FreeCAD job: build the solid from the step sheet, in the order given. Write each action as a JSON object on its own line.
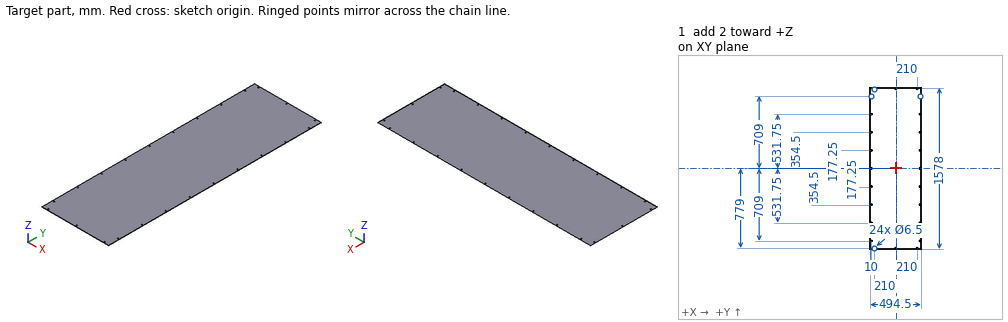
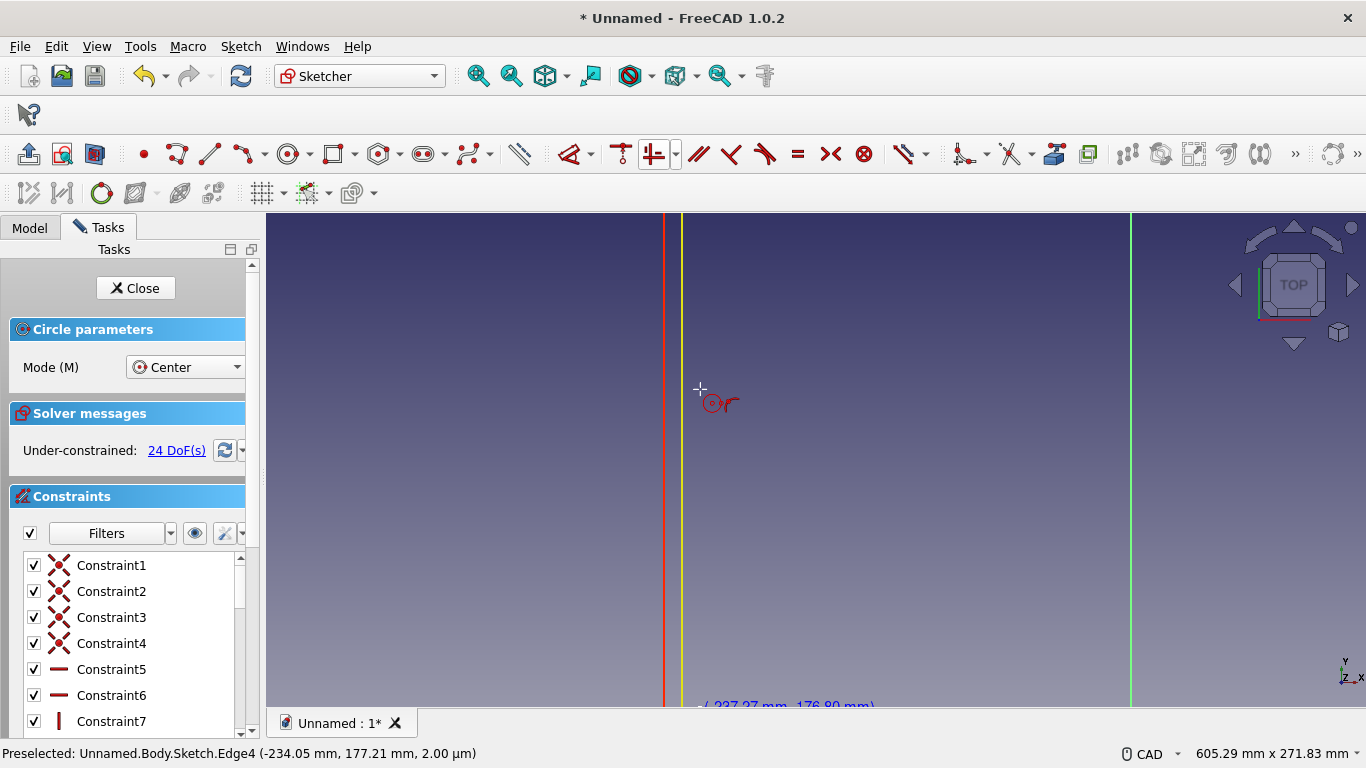
{"action": "left_click", "coordinate": [700, 390]}
{"action": "mouse_move", "coordinate": [704, 385]}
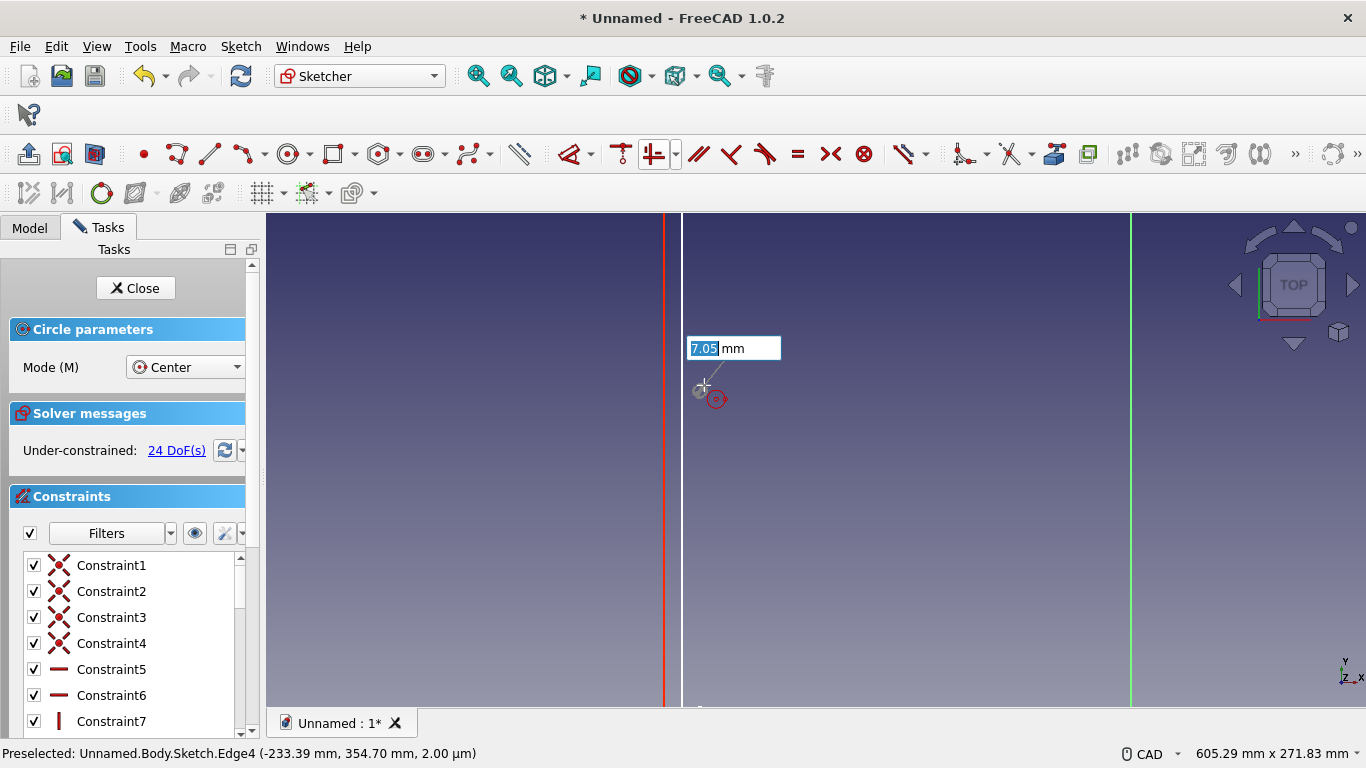
{"action": "type", "text": "6.5"}
{"action": "key", "text": "Return"}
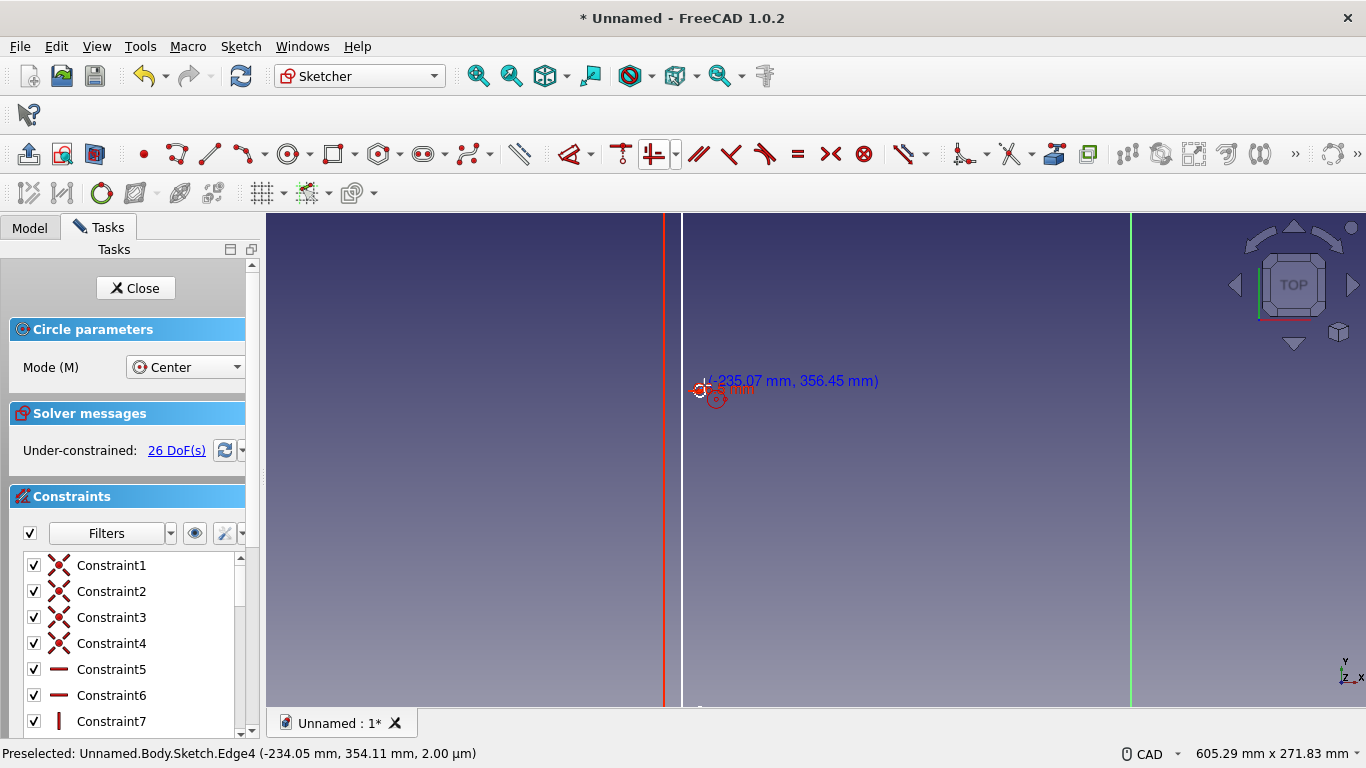
{"action": "scroll", "coordinate": [700, 389], "scroll_direction": "down", "scroll_amount": 11}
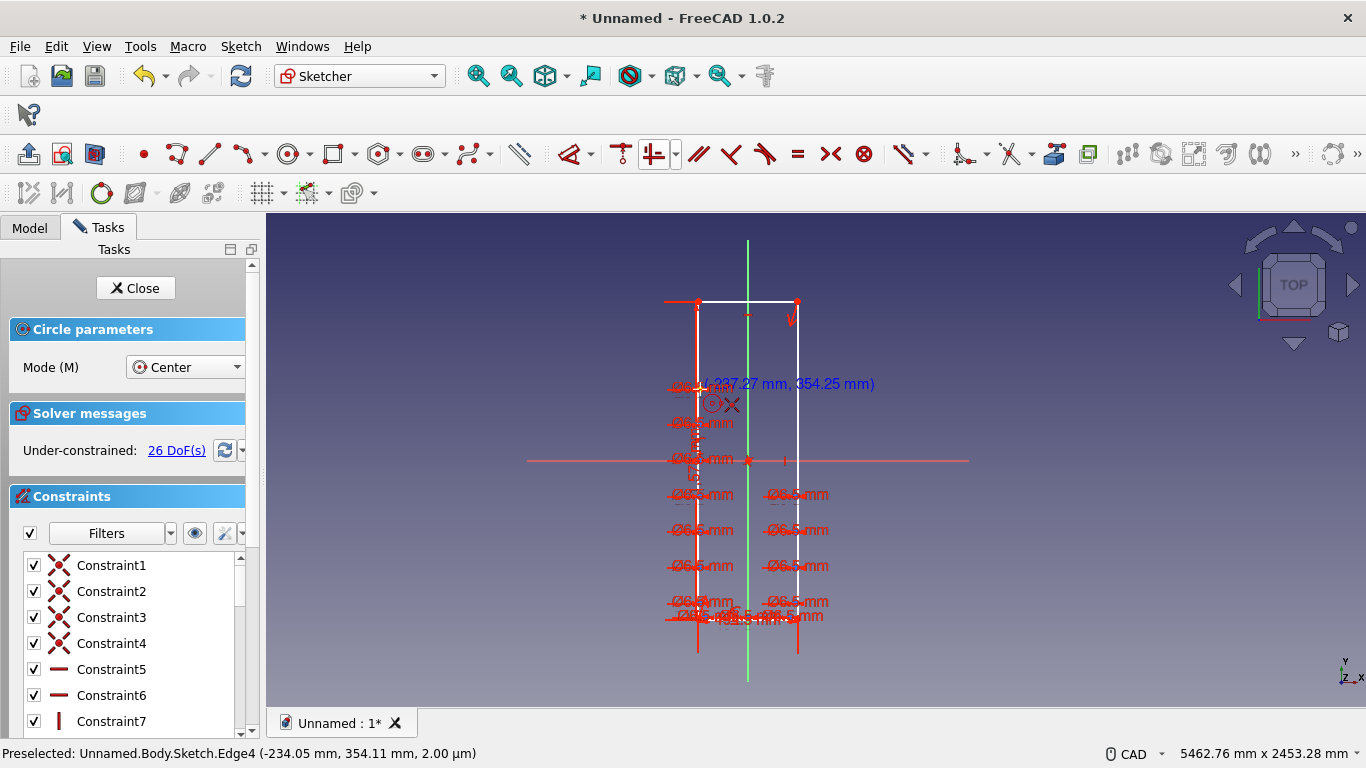
{"action": "scroll", "coordinate": [700, 354], "scroll_direction": "up", "scroll_amount": 18}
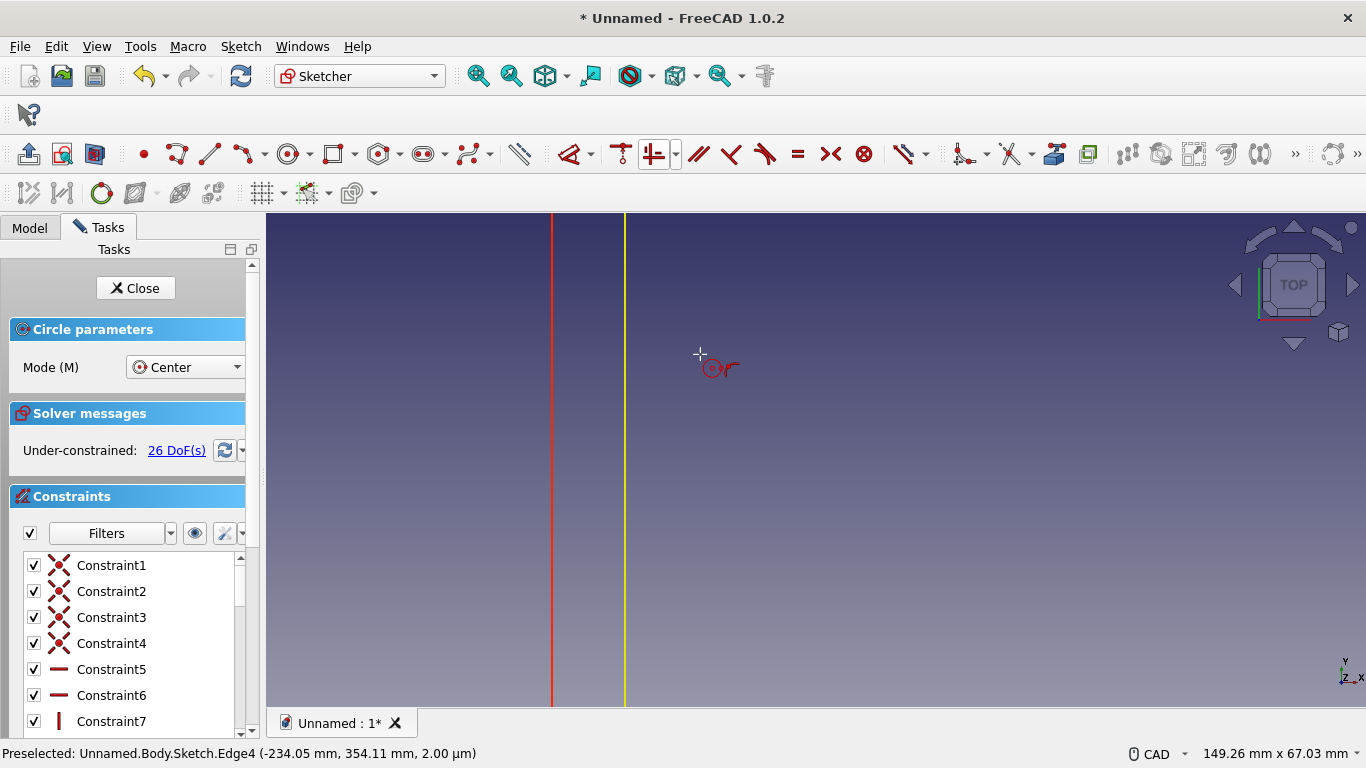
{"action": "scroll", "coordinate": [700, 354], "scroll_direction": "down", "scroll_amount": 18}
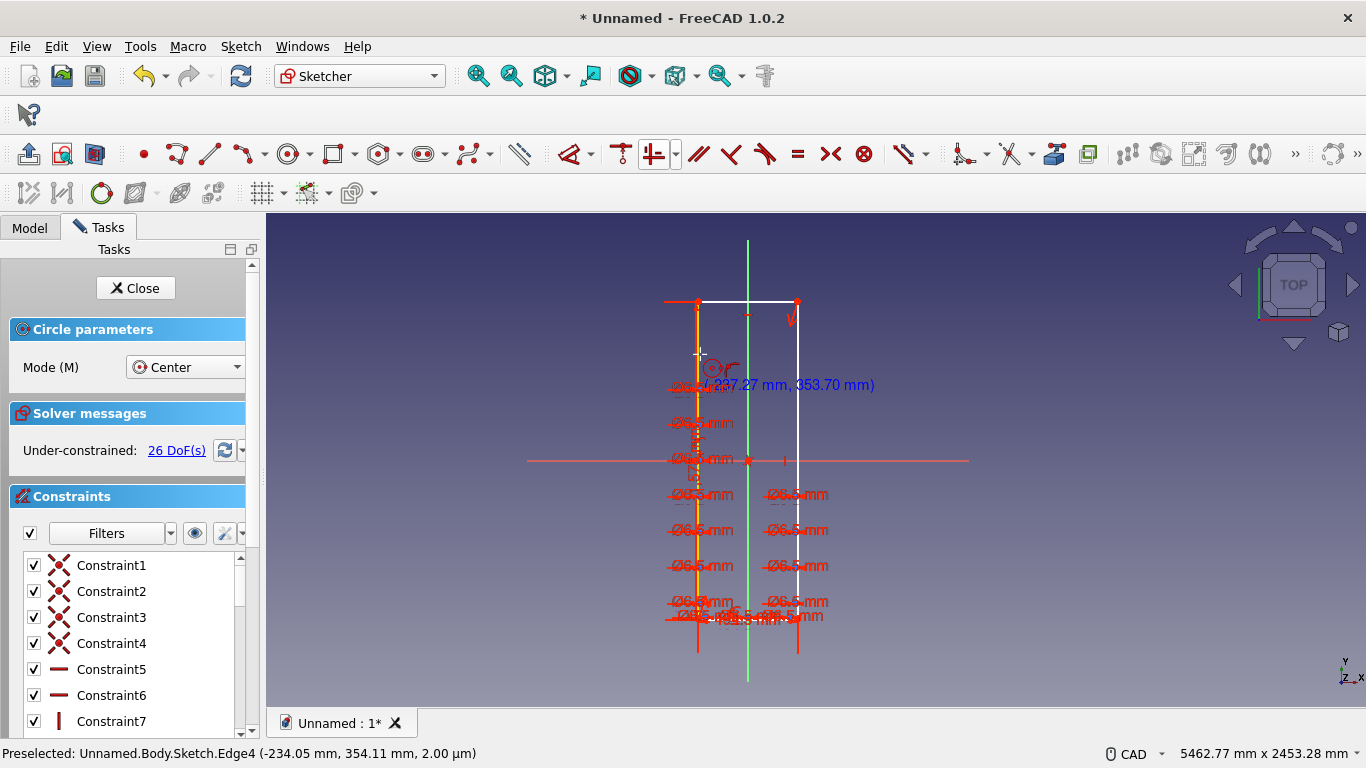
{"action": "scroll", "coordinate": [700, 354], "scroll_direction": "up", "scroll_amount": 11}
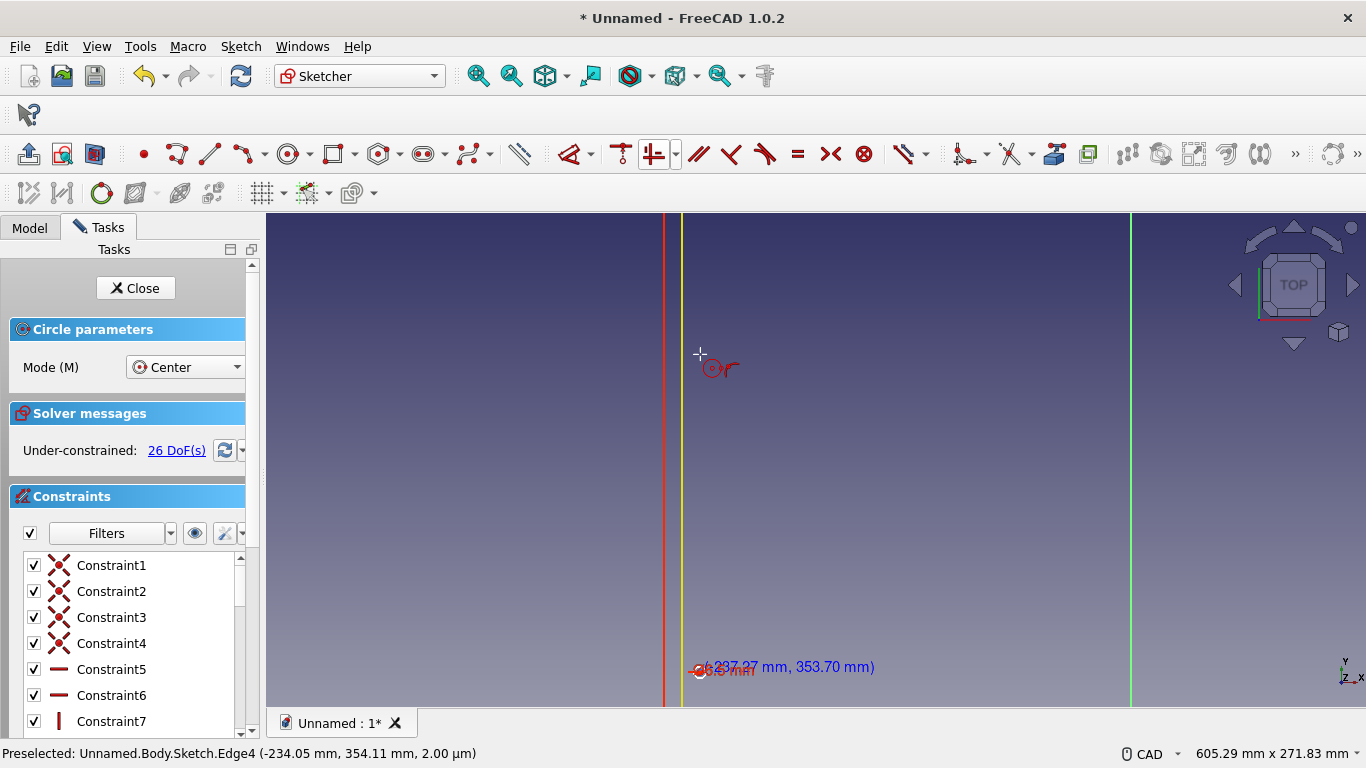
{"action": "left_click", "coordinate": [700, 349]}
{"action": "mouse_move", "coordinate": [704, 345]}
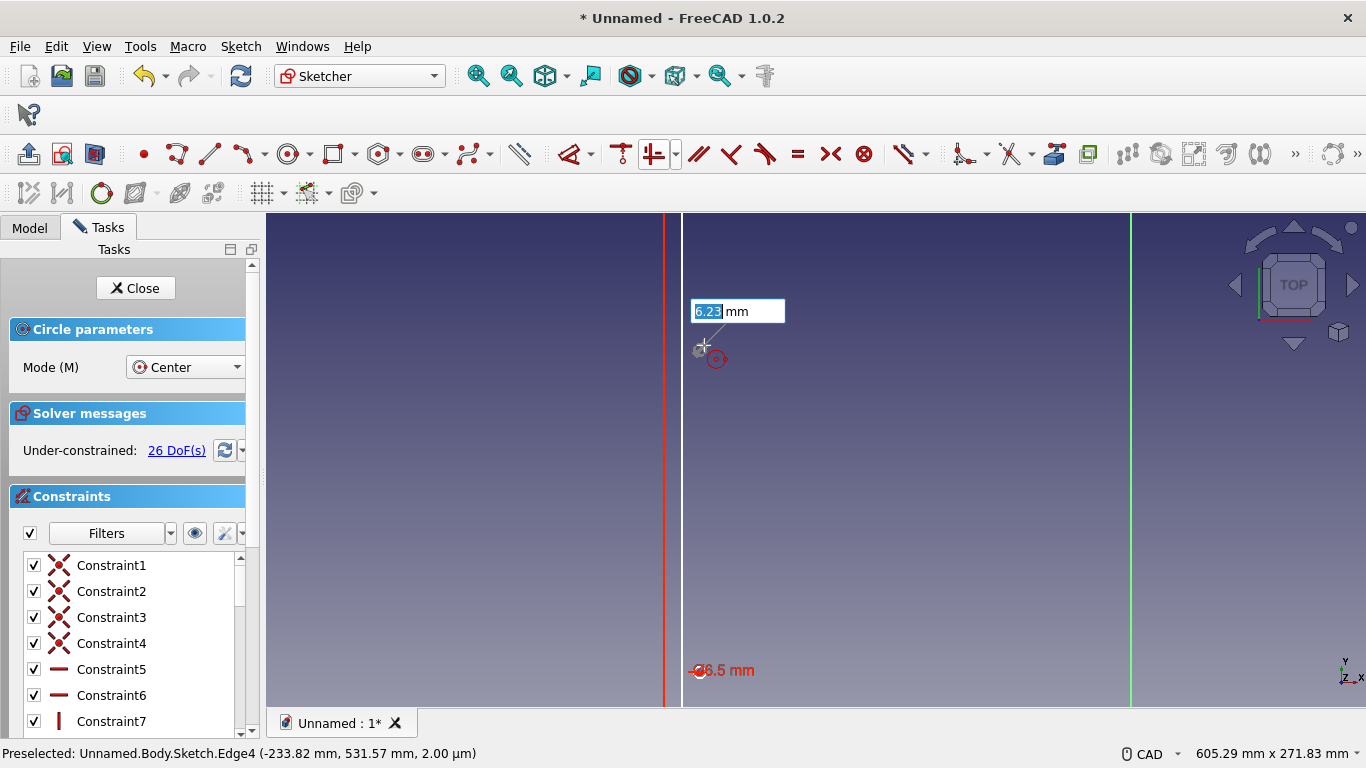
{"action": "type", "text": "6.5"}
{"action": "key", "text": "Return"}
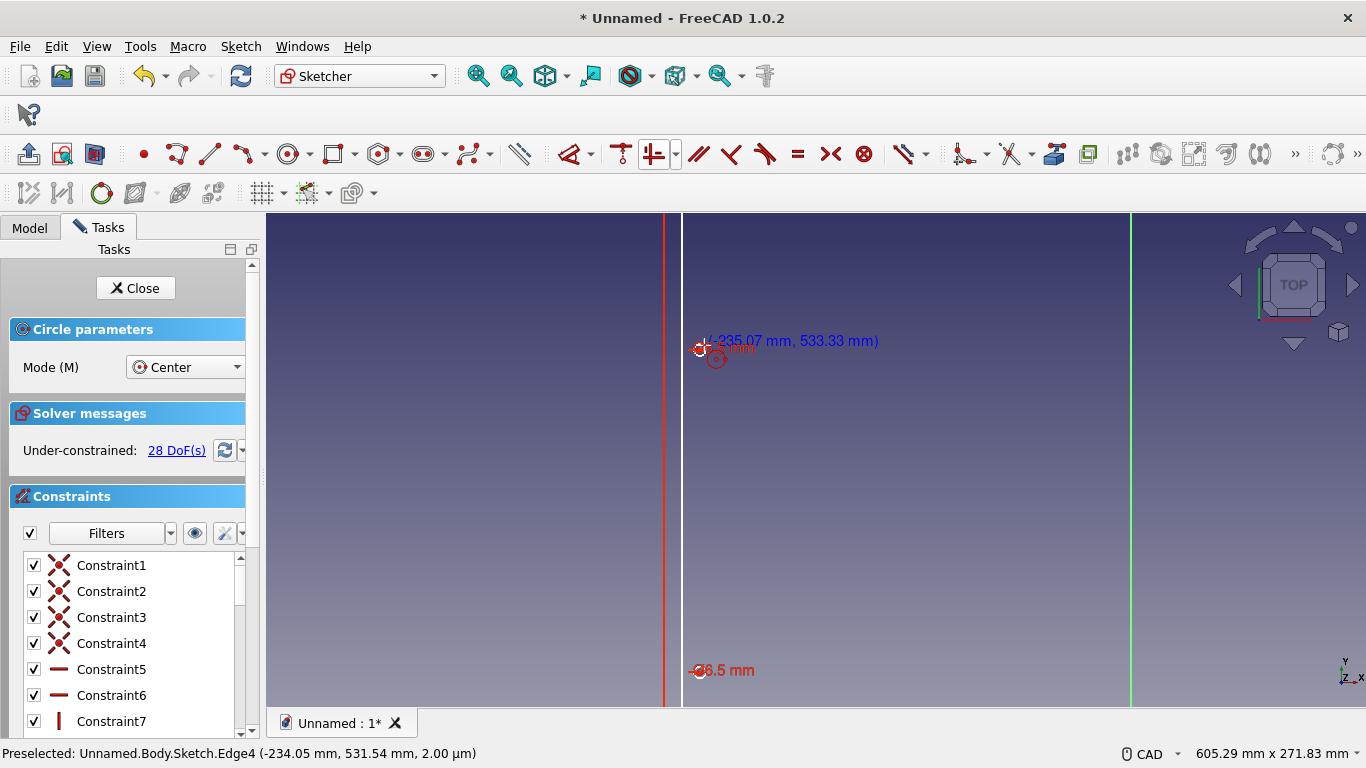
{"action": "scroll", "coordinate": [700, 353], "scroll_direction": "down", "scroll_amount": 11}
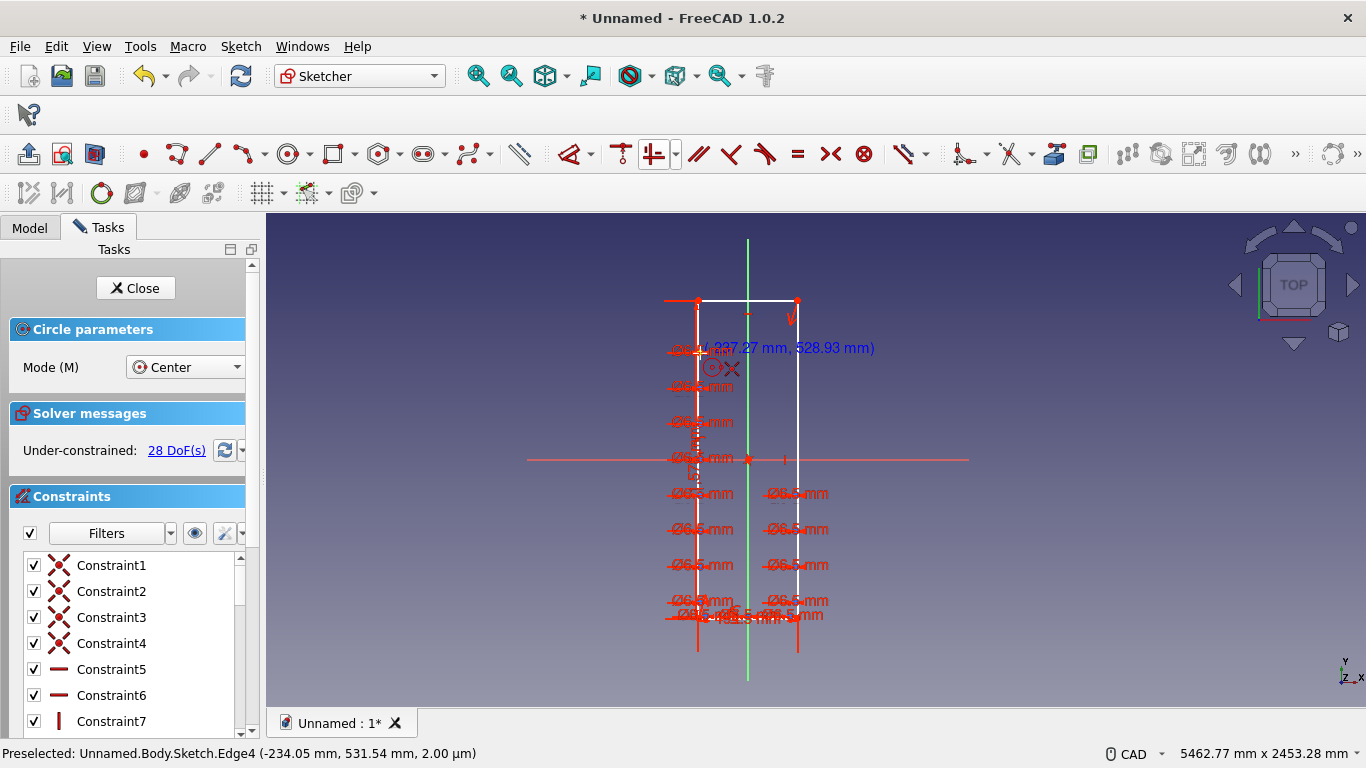
{"action": "scroll", "coordinate": [700, 317], "scroll_direction": "up", "scroll_amount": 18}